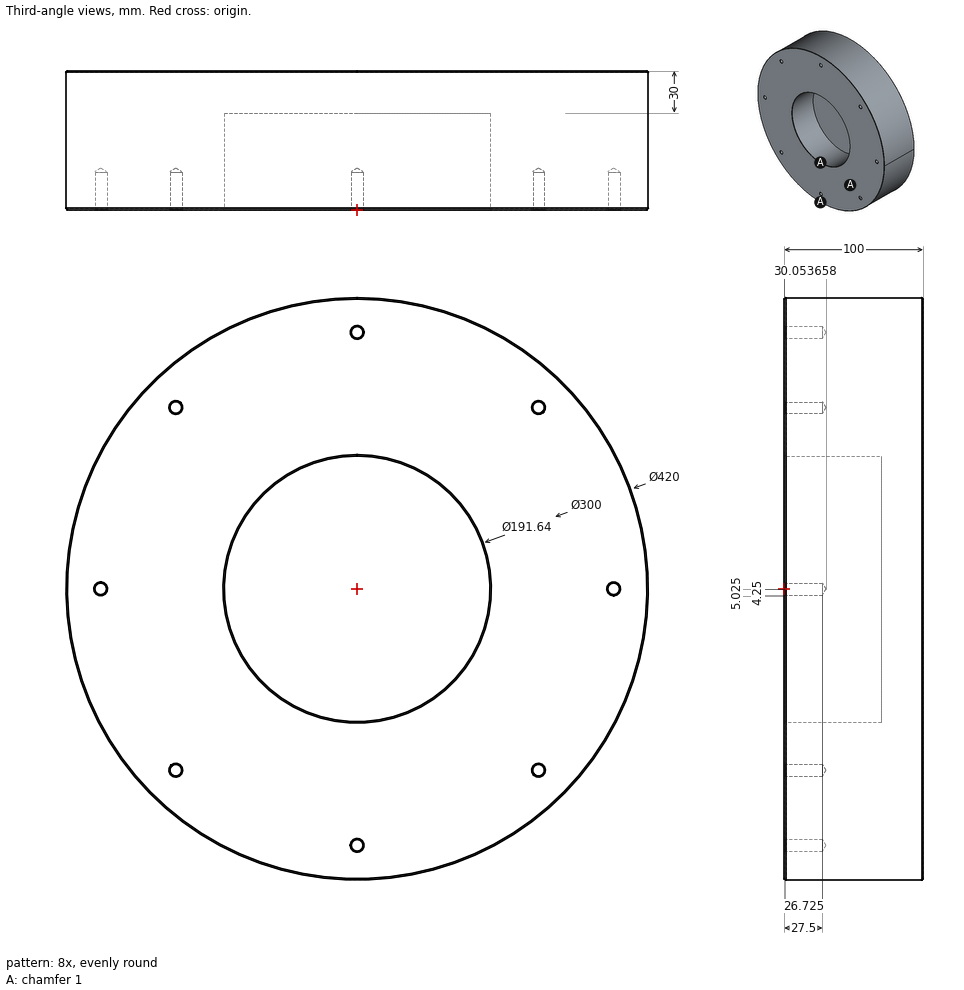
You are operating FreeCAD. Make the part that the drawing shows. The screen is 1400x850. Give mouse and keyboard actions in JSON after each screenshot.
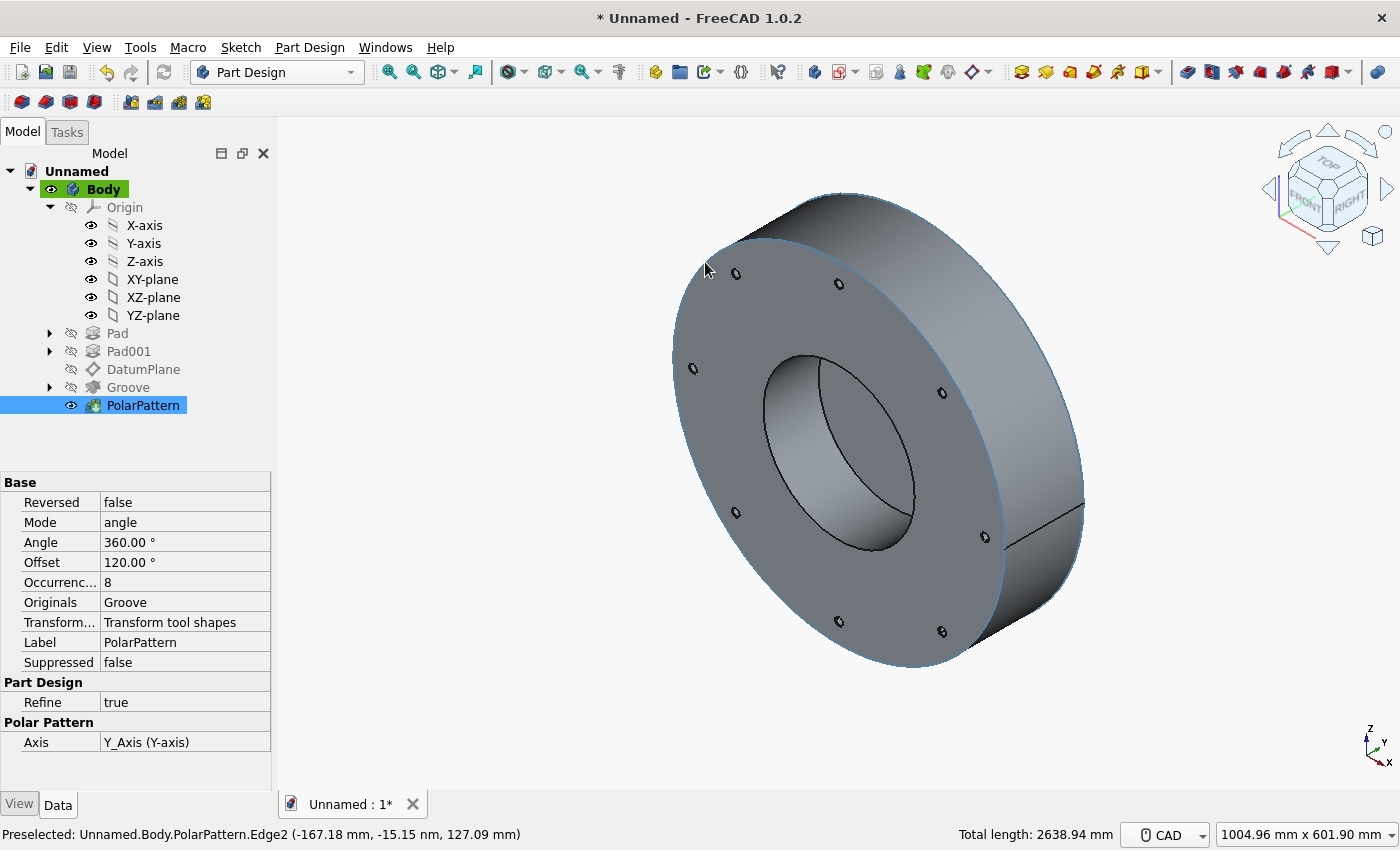
{"action": "left_click", "coordinate": [763, 408], "text": "ctrl"}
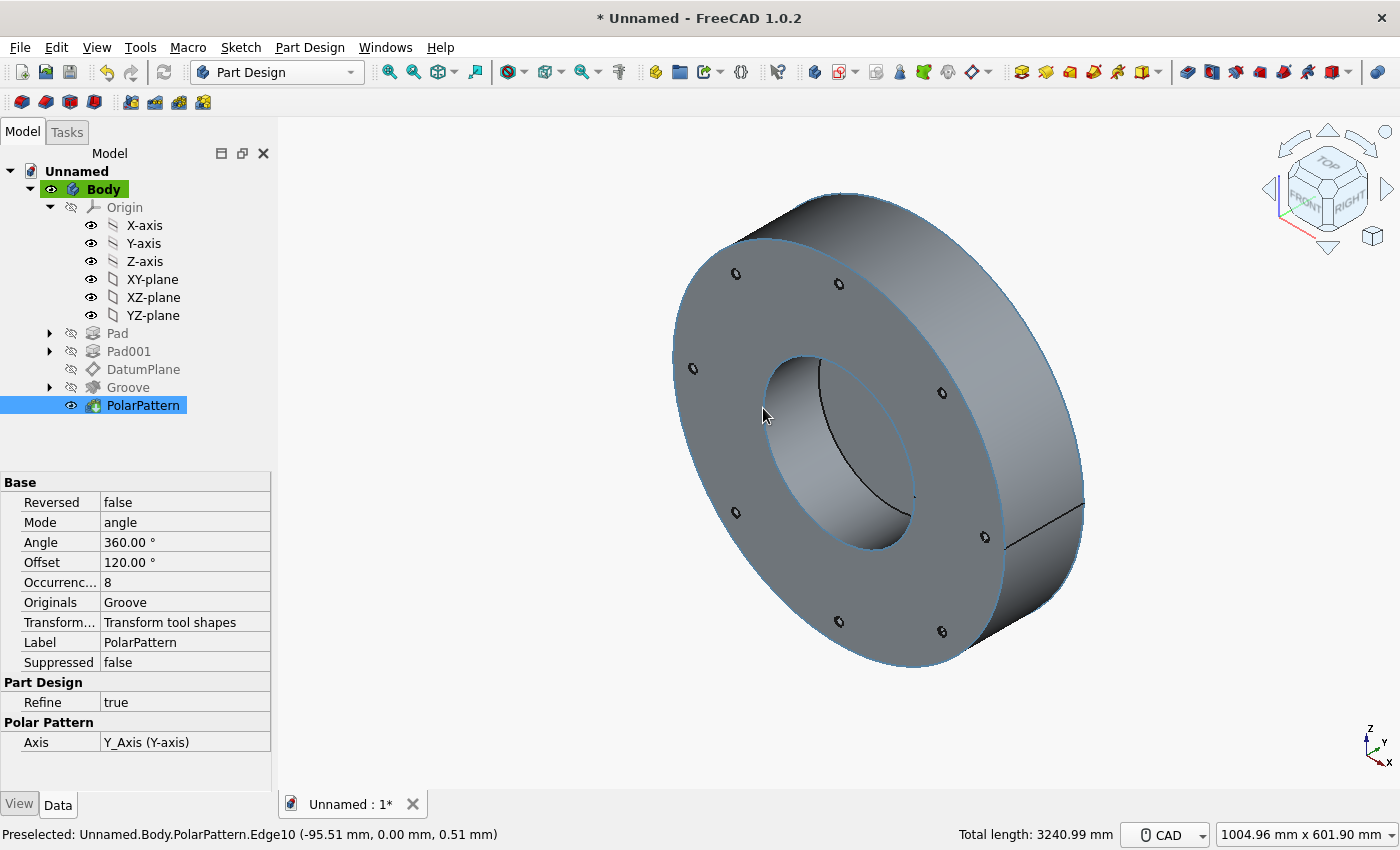
{"action": "left_click", "coordinate": [46, 102]}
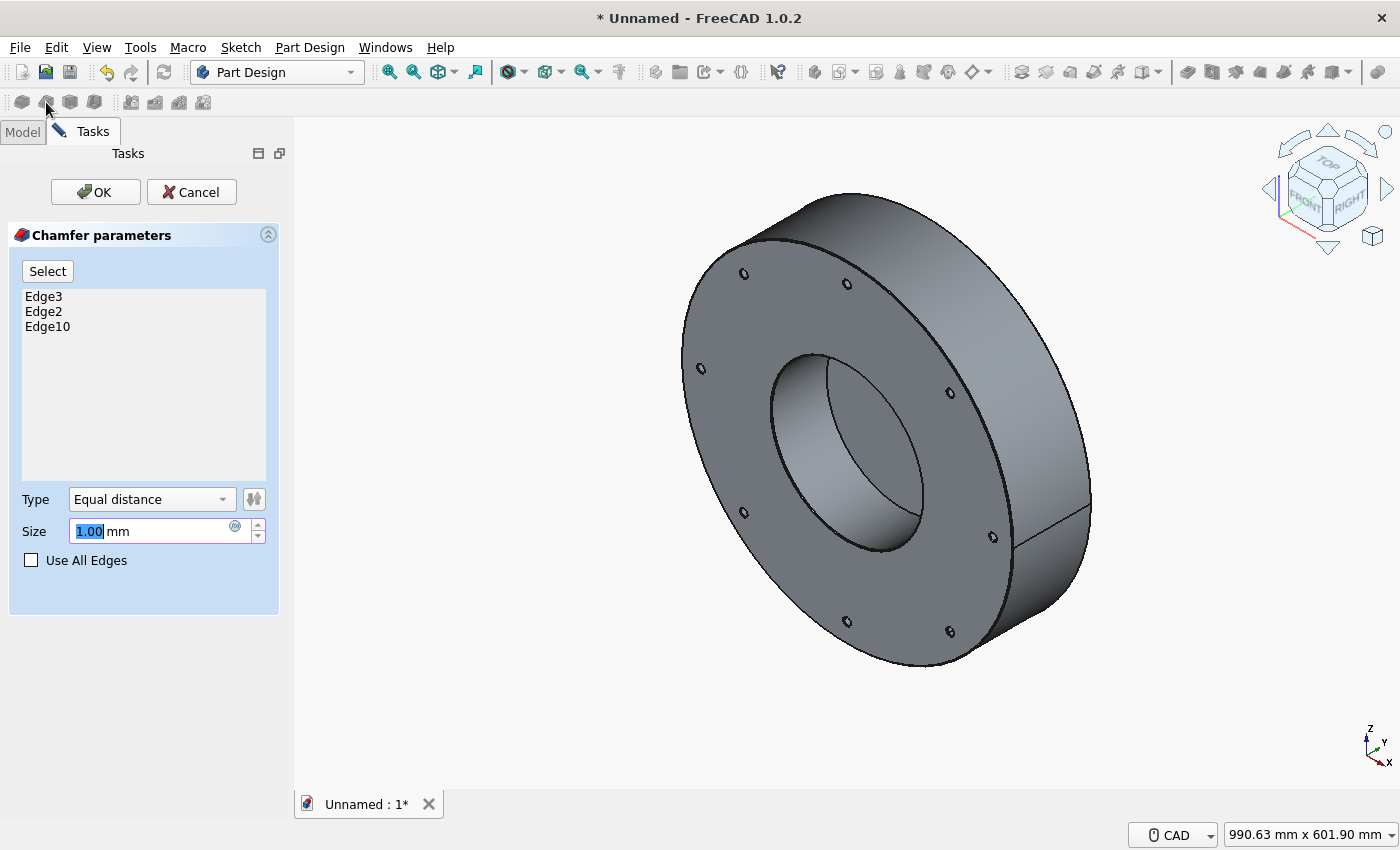
{"action": "type", "text": "1"}
{"action": "key", "text": "Tab"}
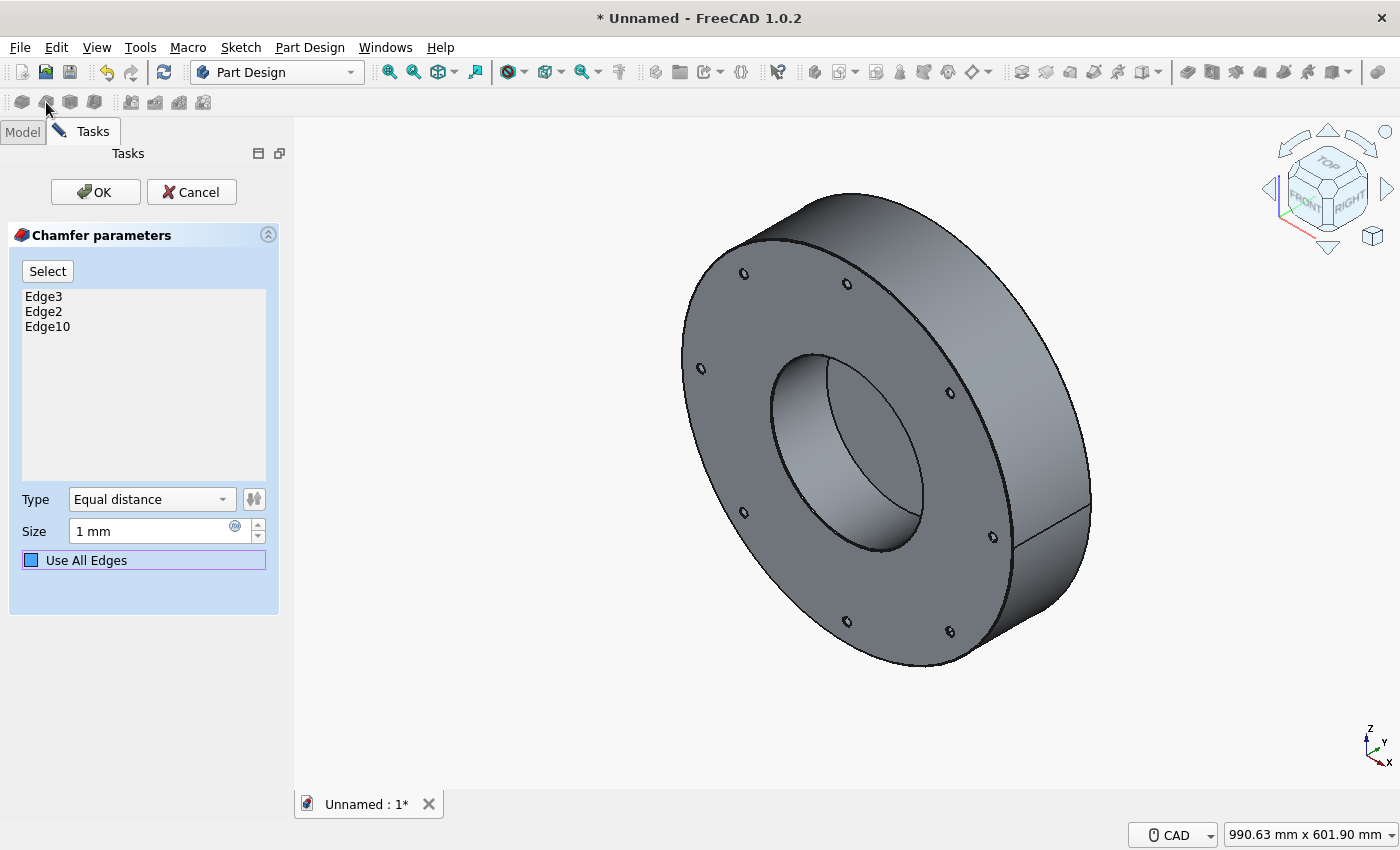
{"action": "left_click", "coordinate": [96, 192]}